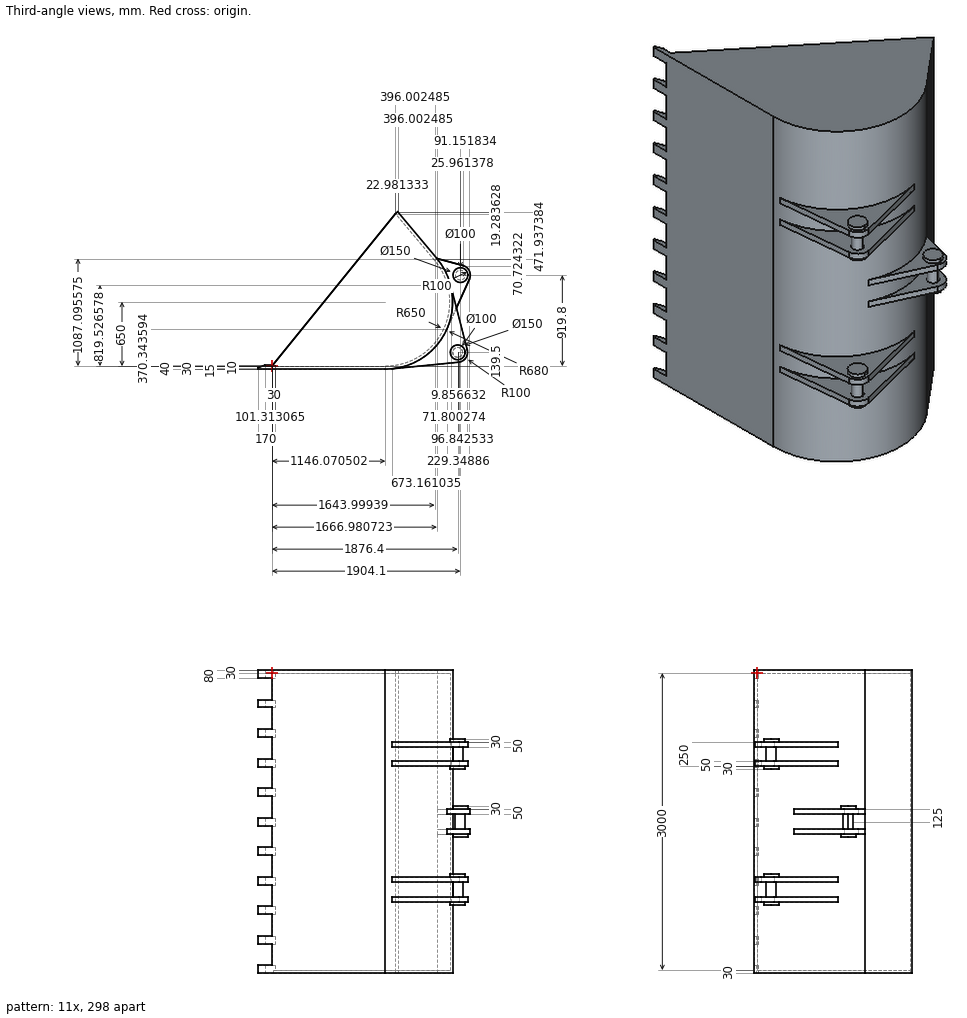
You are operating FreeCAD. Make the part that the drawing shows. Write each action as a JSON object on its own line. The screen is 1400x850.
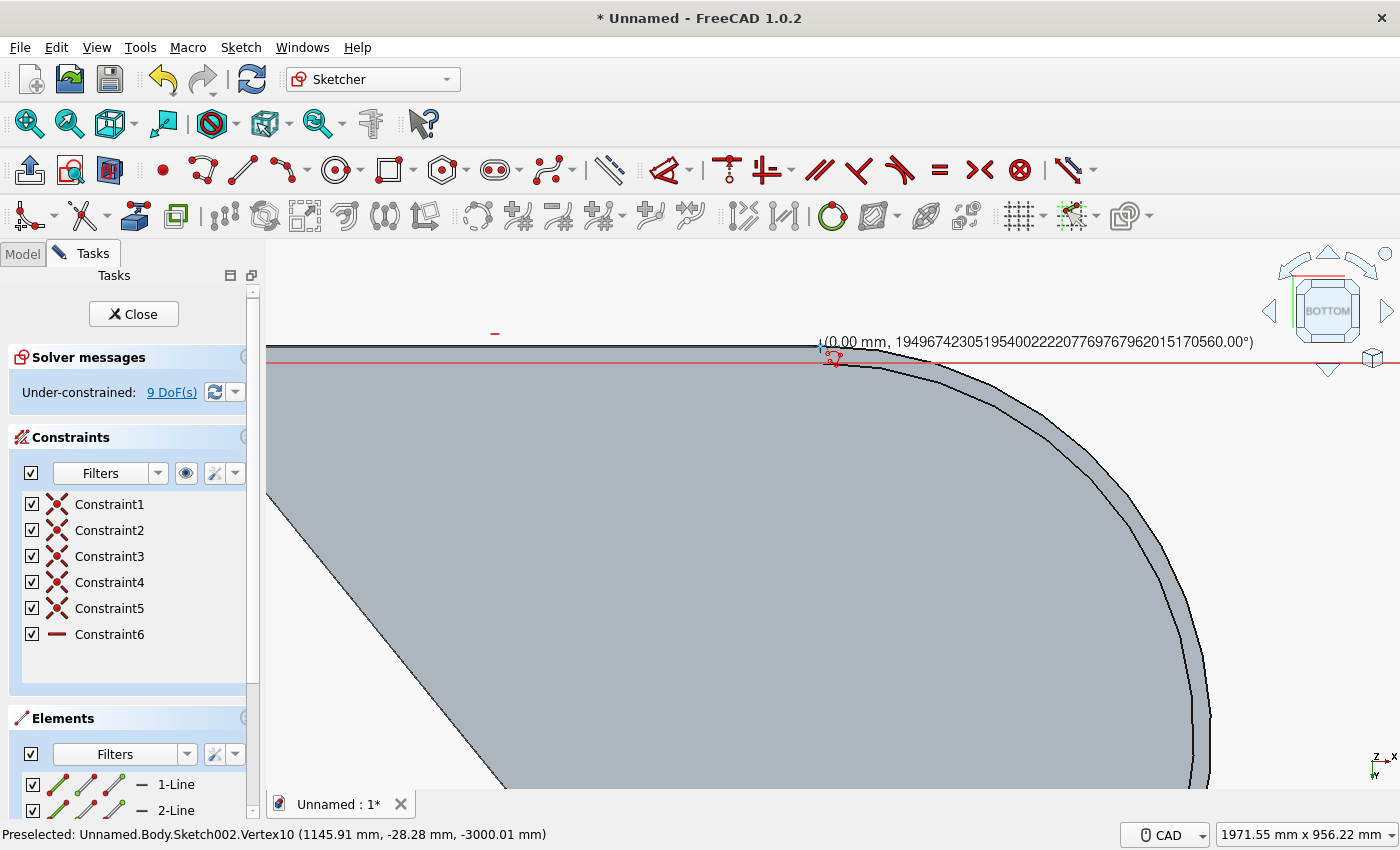
{"action": "left_click", "coordinate": [284, 170]}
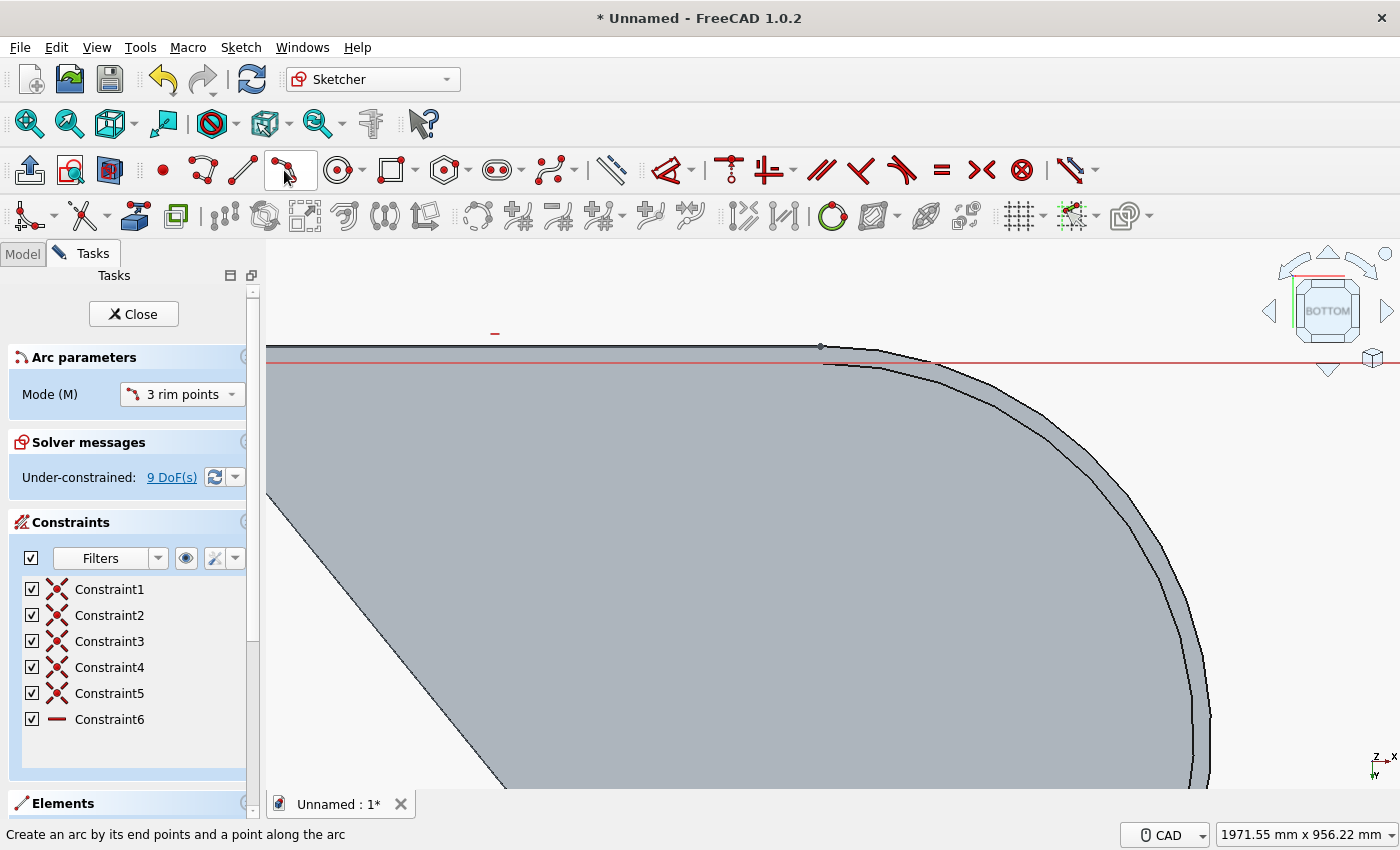
{"action": "left_click", "coordinate": [820, 347]}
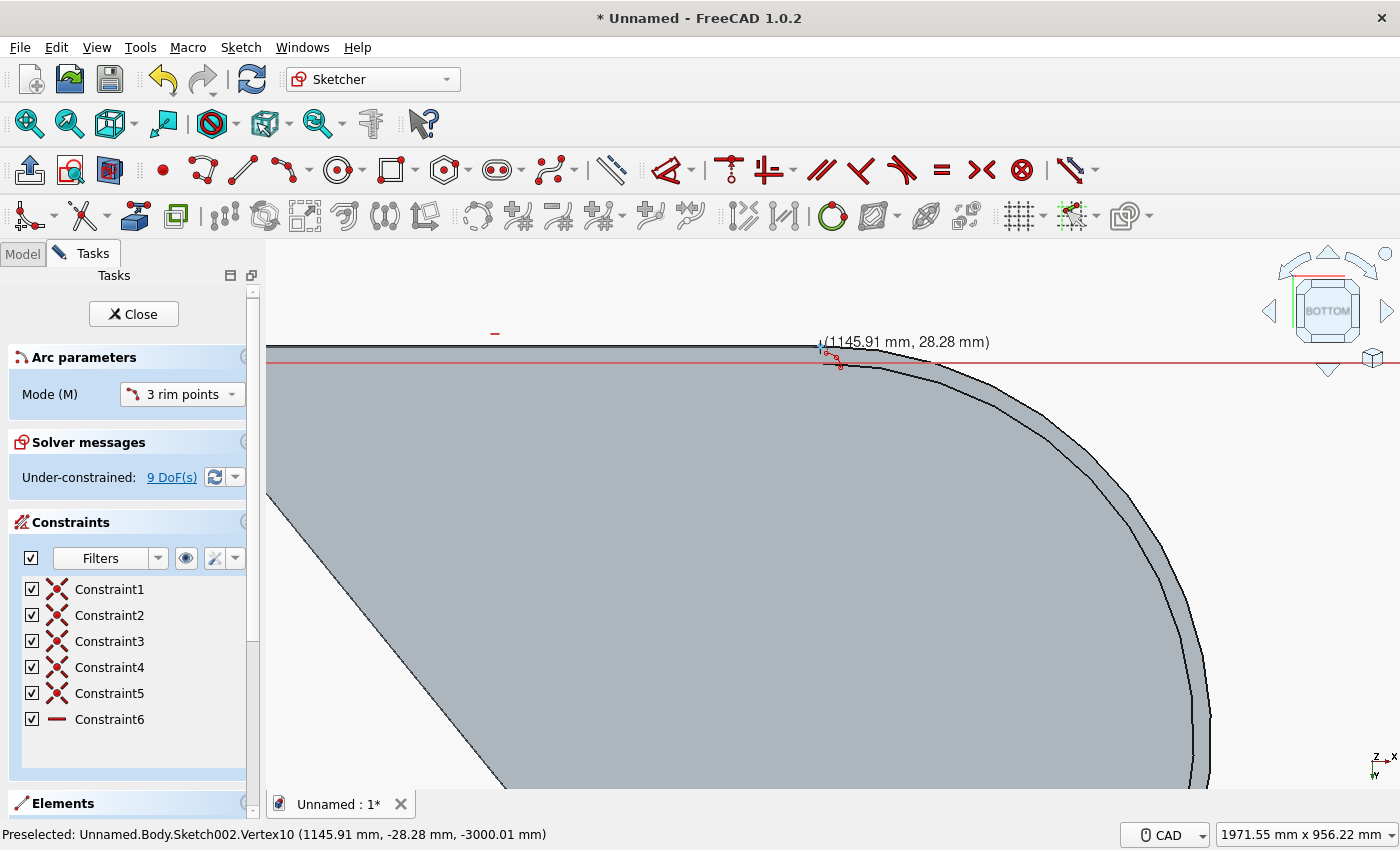
{"action": "scroll", "coordinate": [821, 346], "scroll_direction": "down", "scroll_amount": 5}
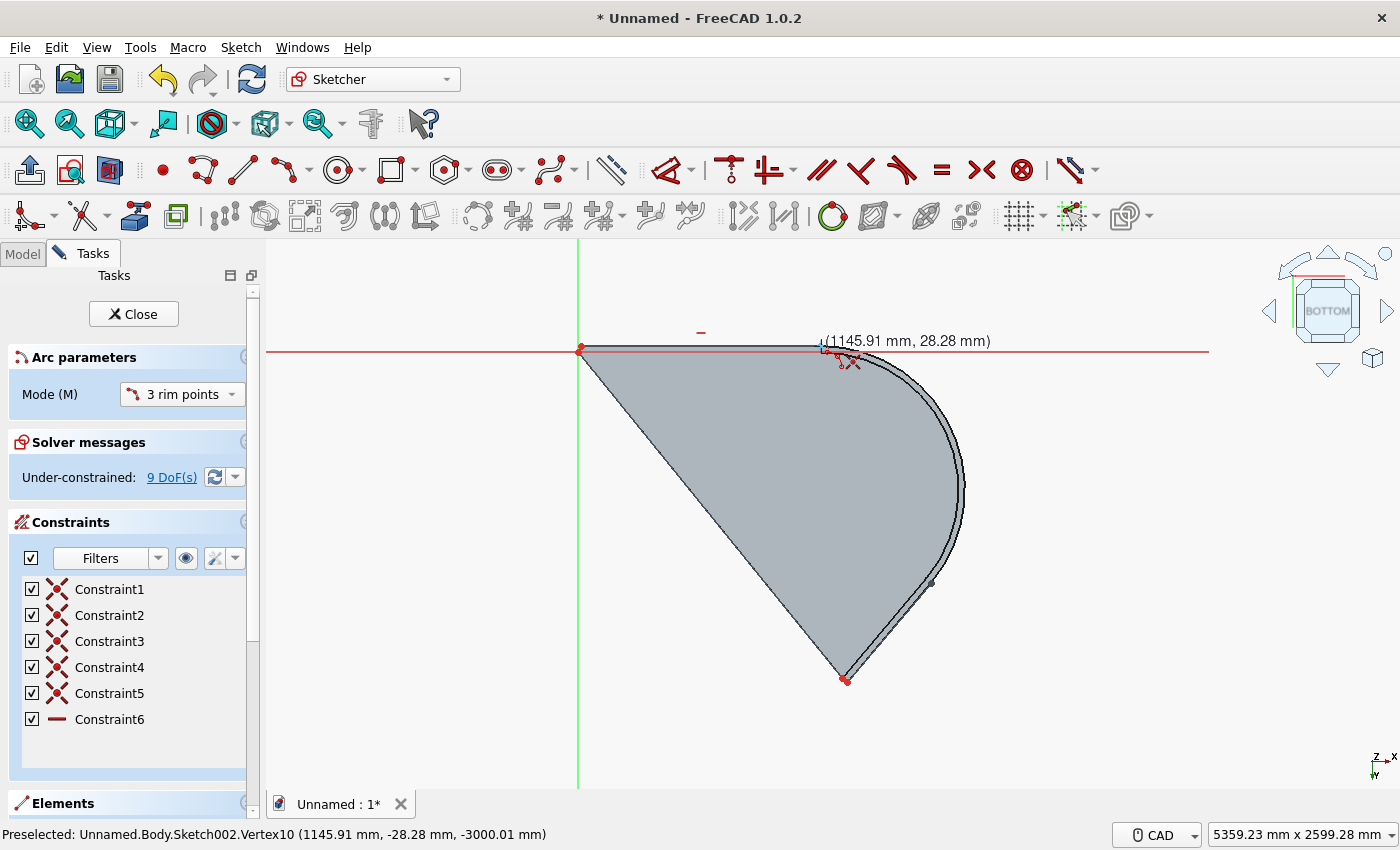
{"action": "left_click", "coordinate": [931, 584]}
{"action": "left_click", "coordinate": [951, 429]}
{"action": "key", "text": "Escape"}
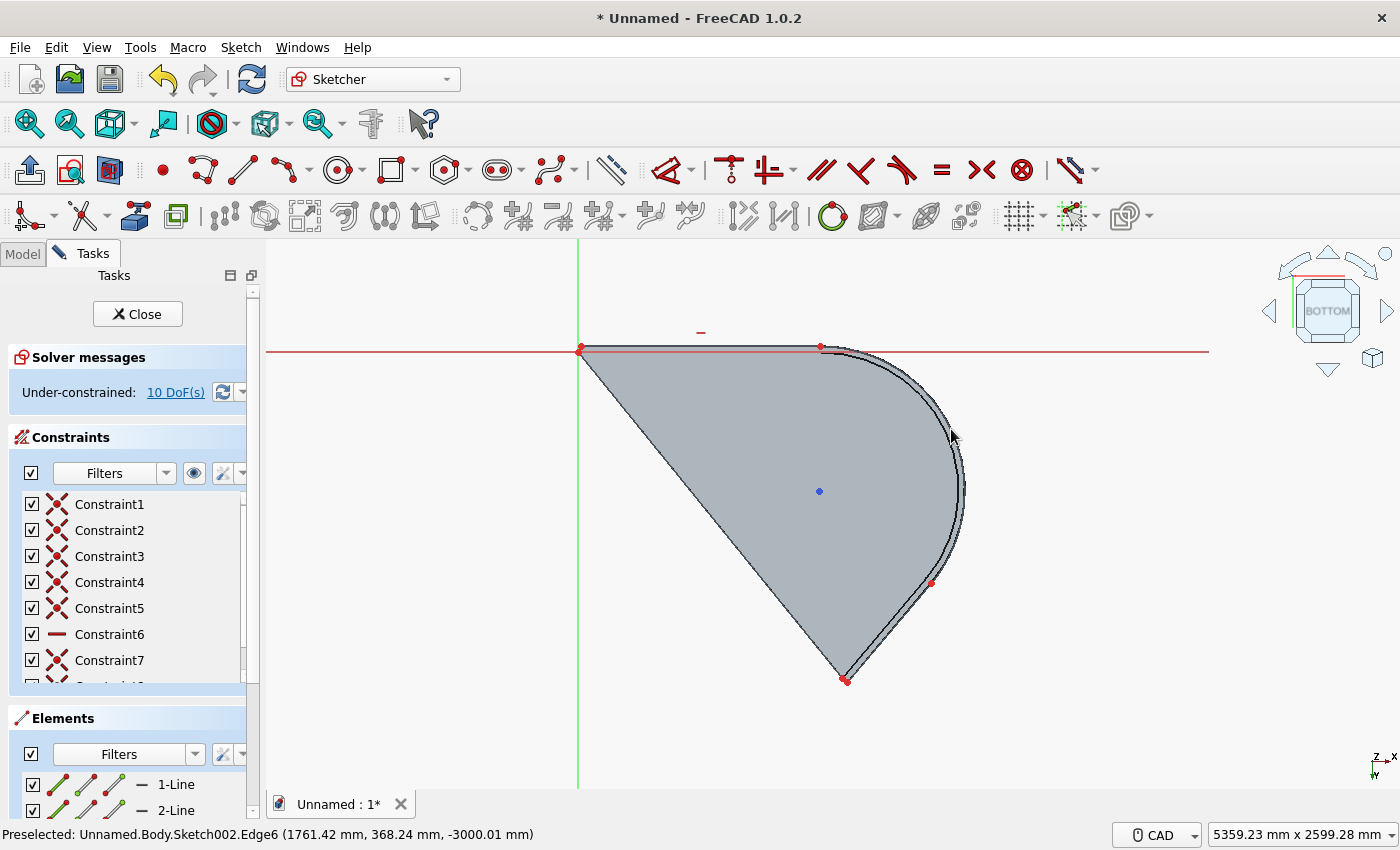
{"action": "scroll", "coordinate": [580, 349], "scroll_direction": "up", "scroll_amount": 7}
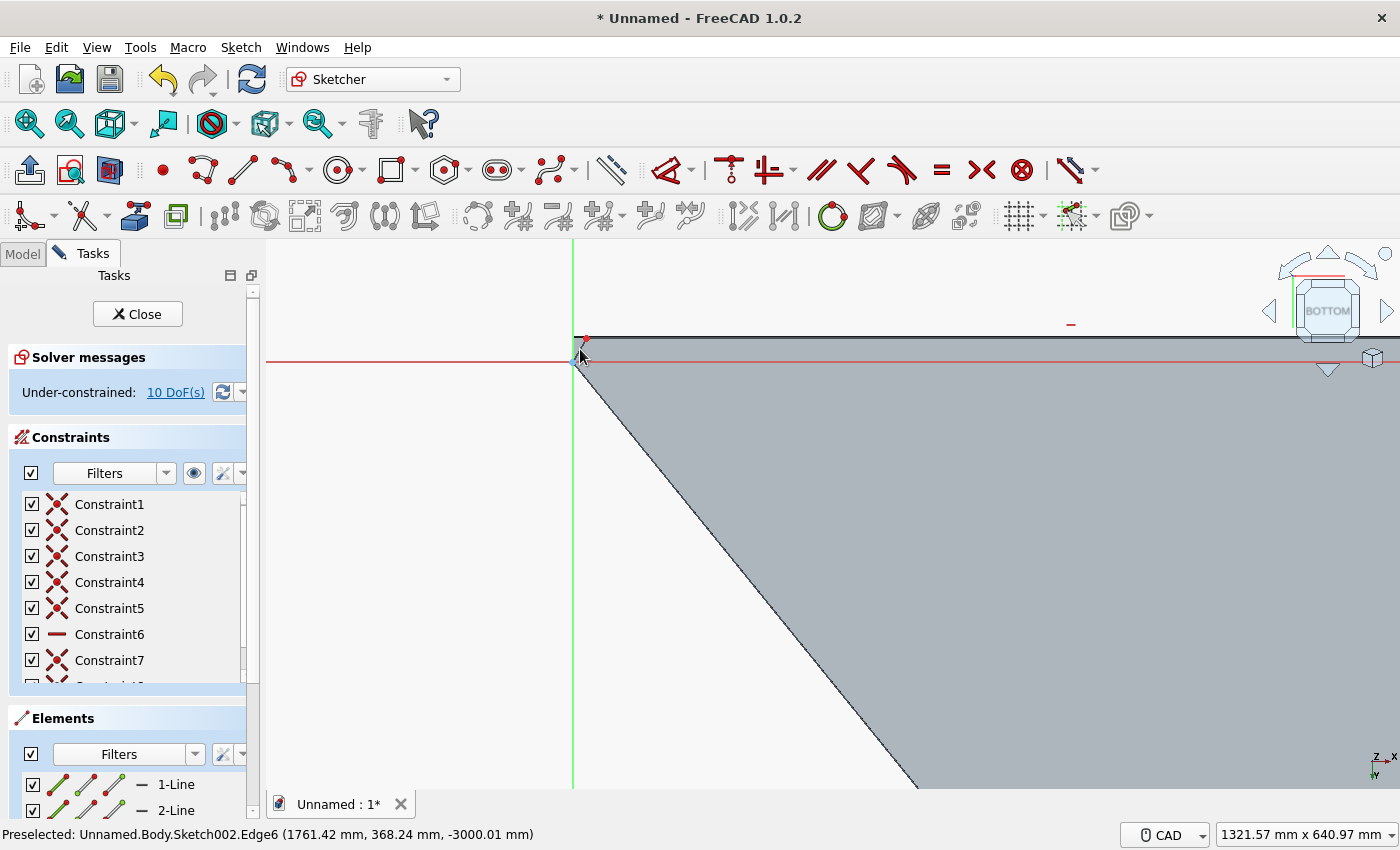
{"action": "left_click", "coordinate": [580, 350]}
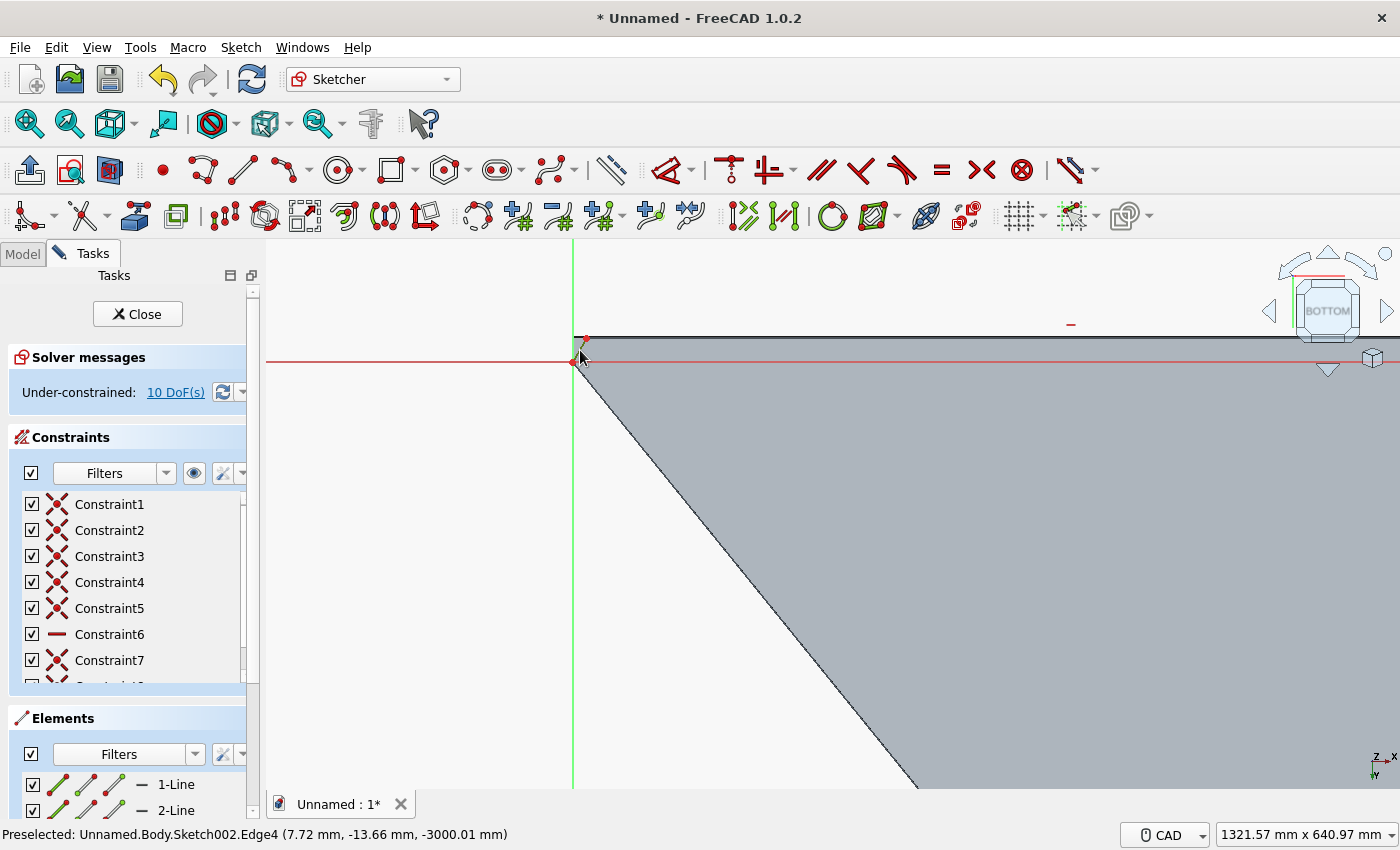
{"action": "left_click", "coordinate": [796, 170]}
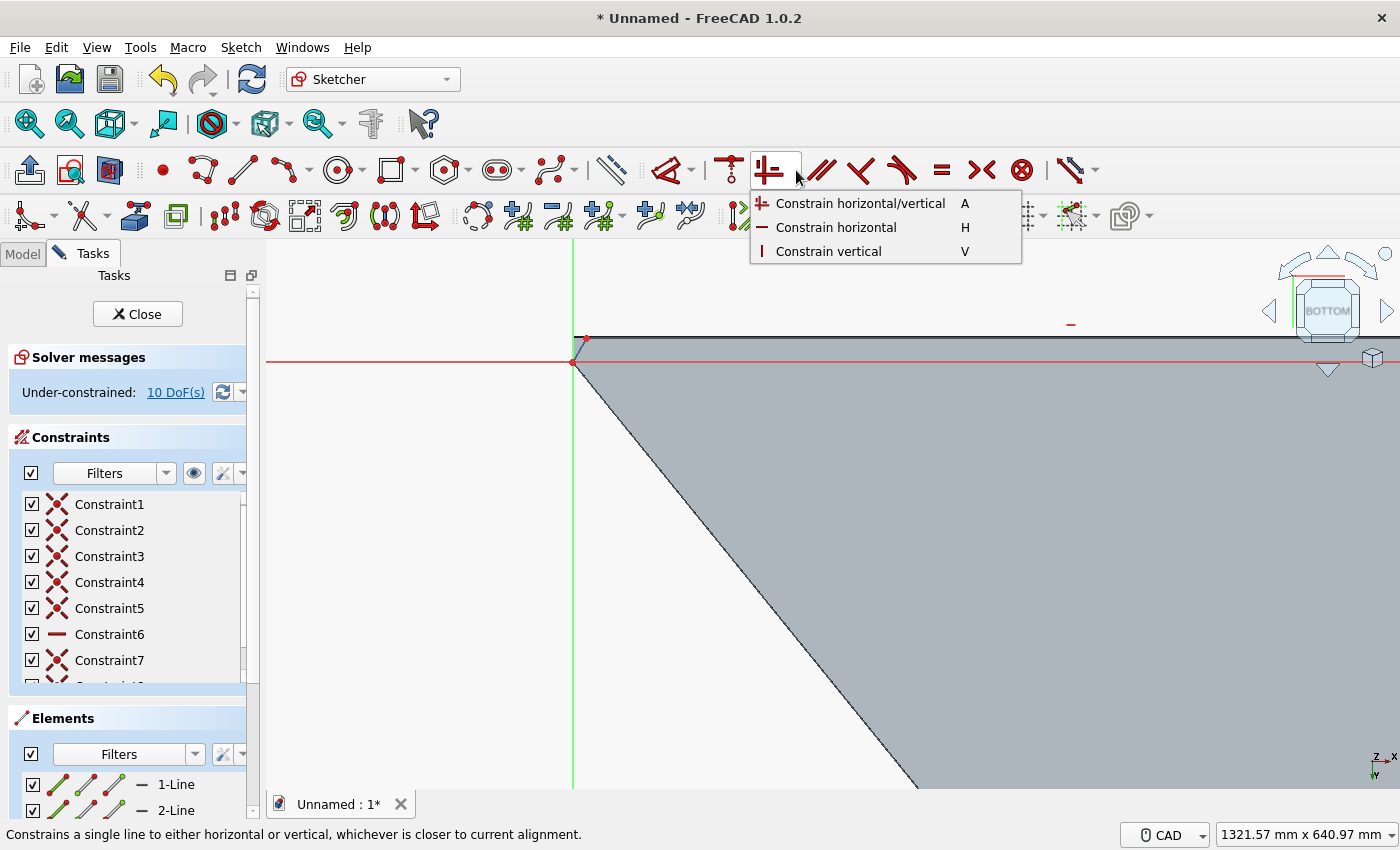
{"action": "left_click", "coordinate": [886, 251]}